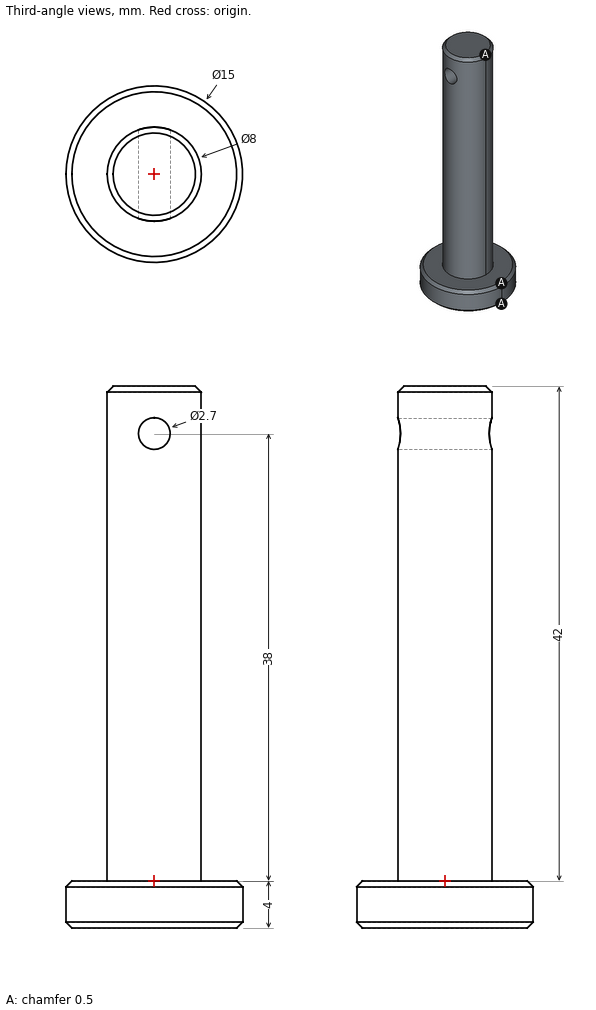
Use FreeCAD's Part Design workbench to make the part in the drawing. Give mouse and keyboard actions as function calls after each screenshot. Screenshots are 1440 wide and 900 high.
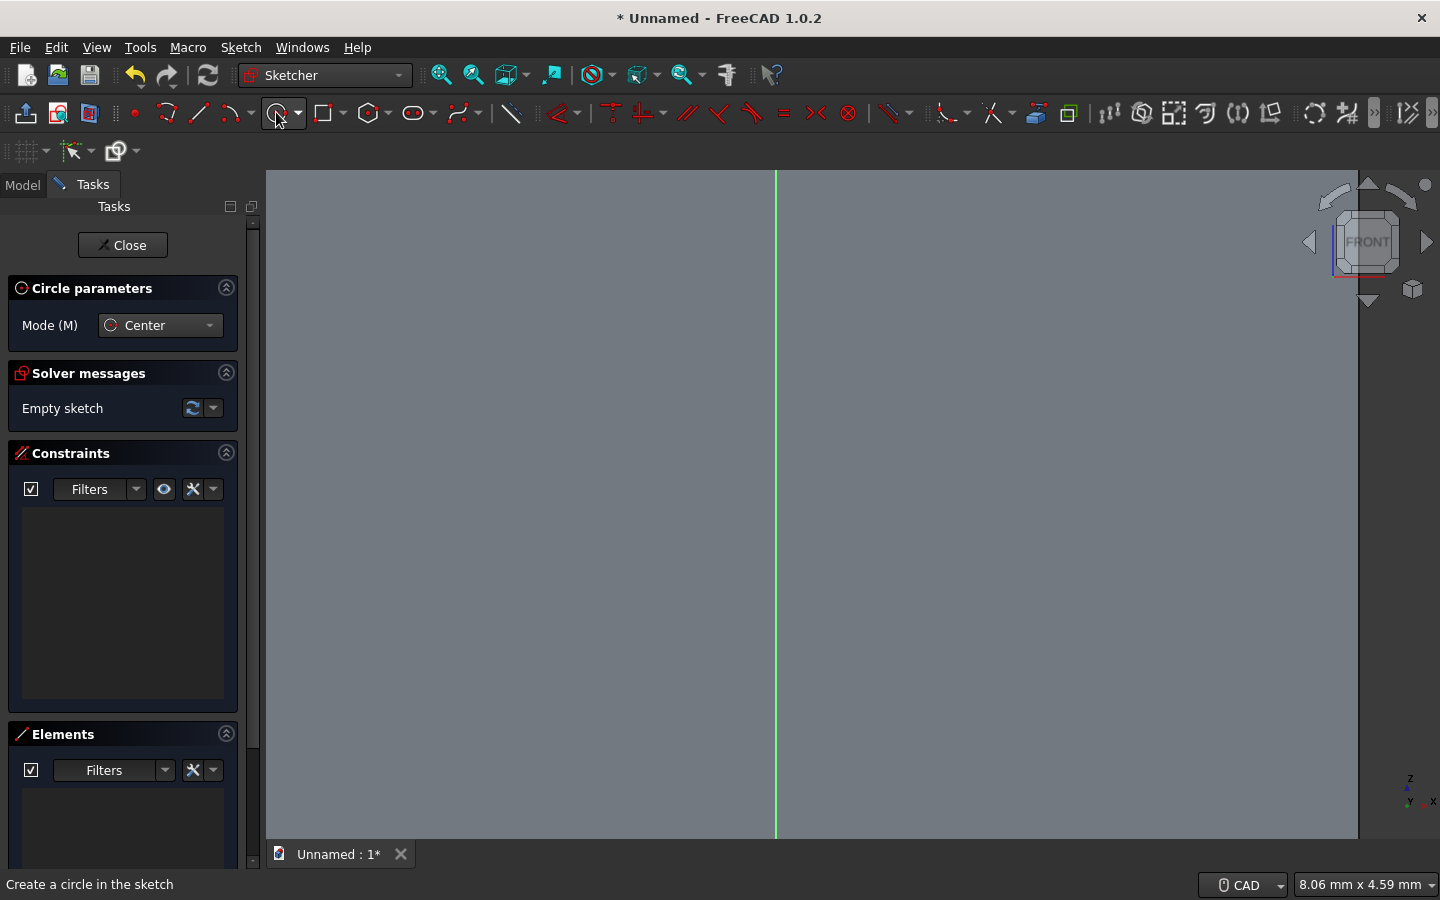
click(776, 500)
move(915, 361)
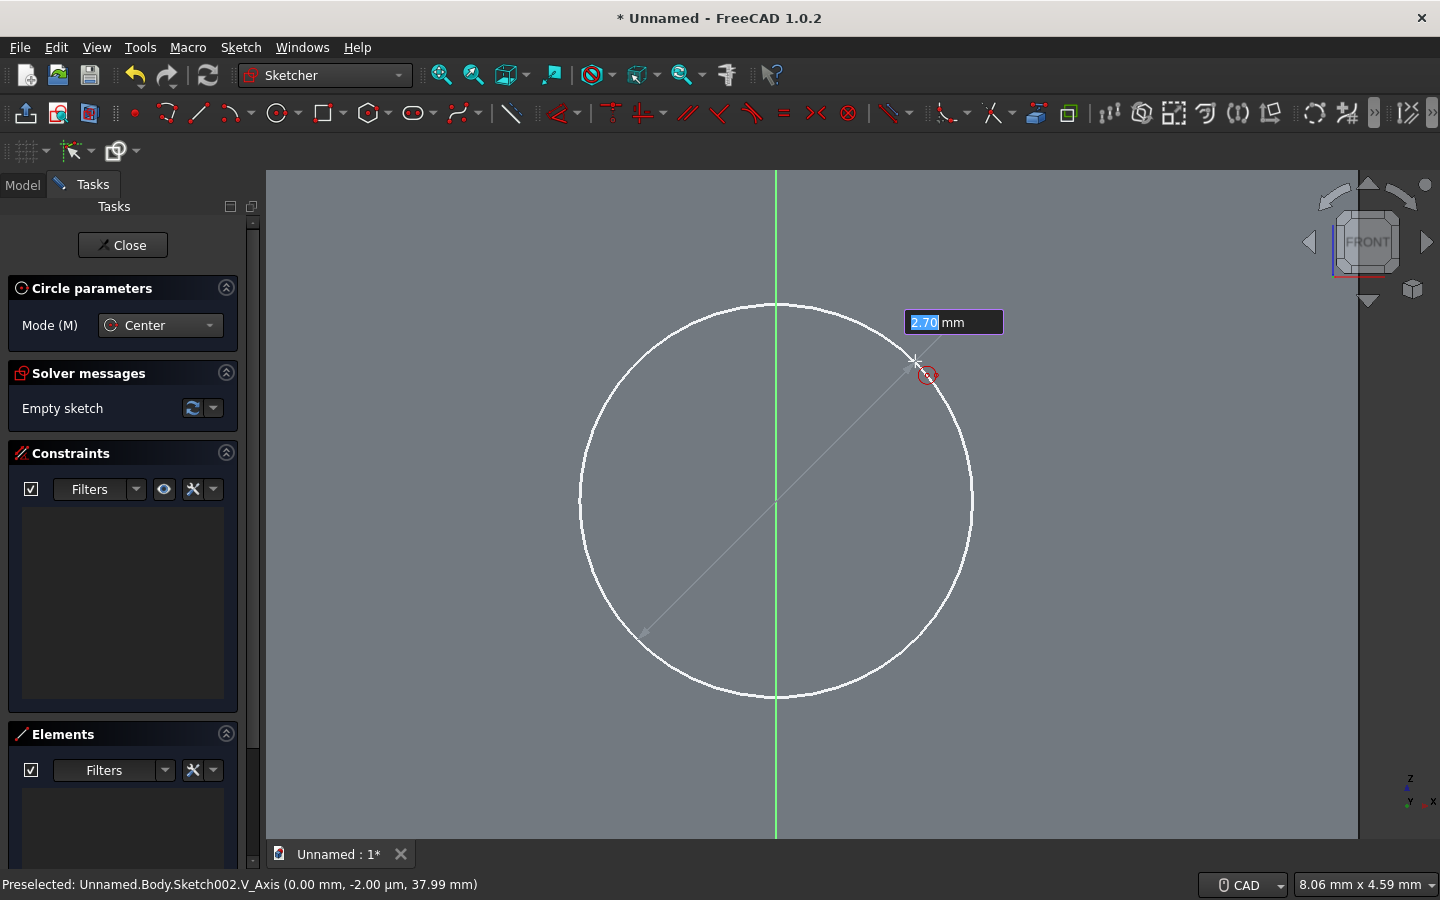
text(2.7)
key(Return)
key(Escape)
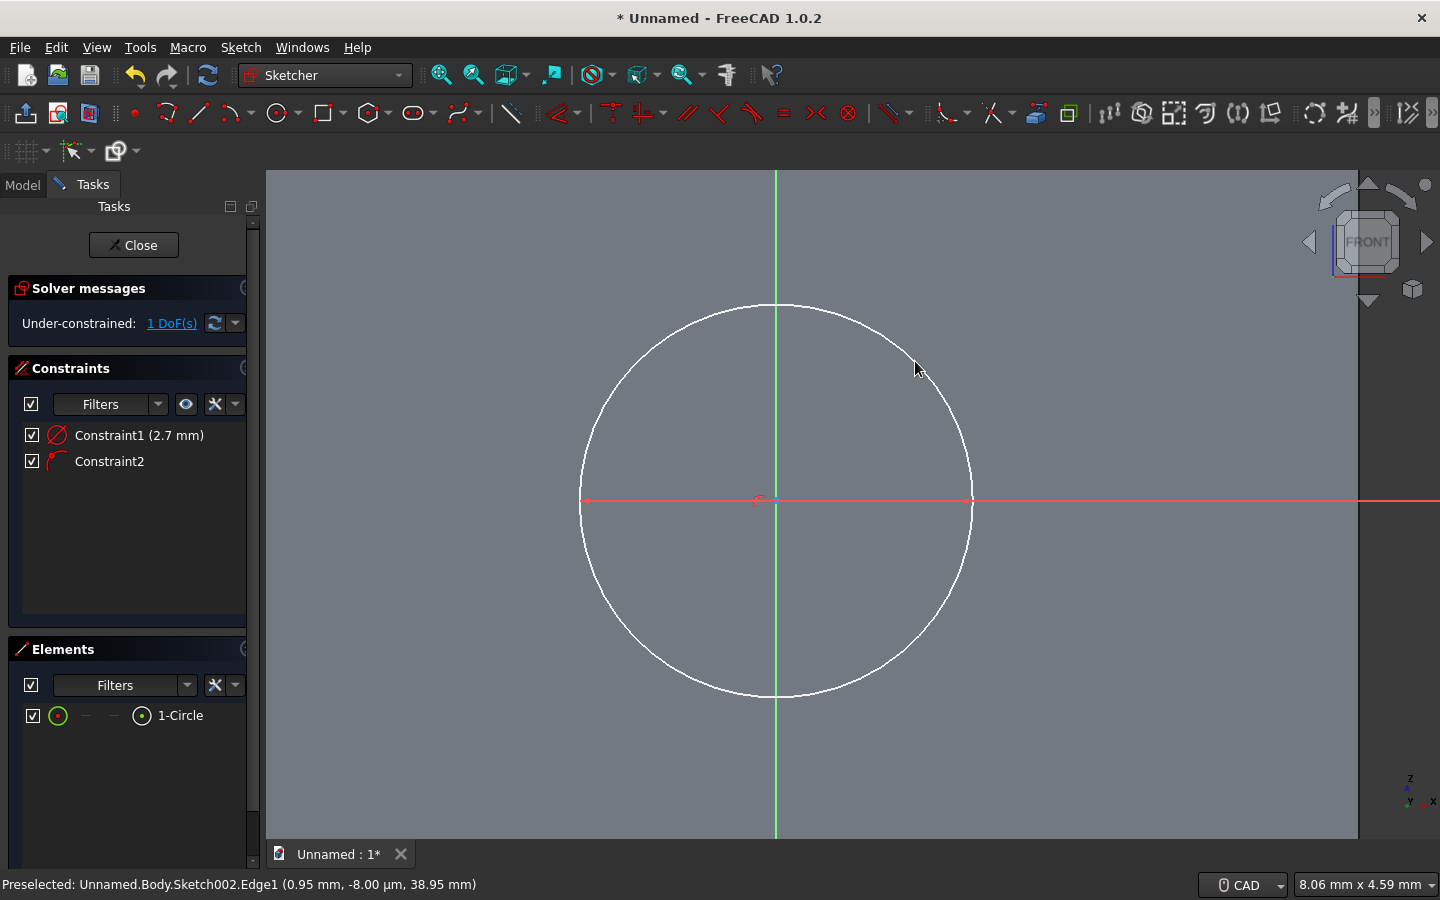
click(776, 501)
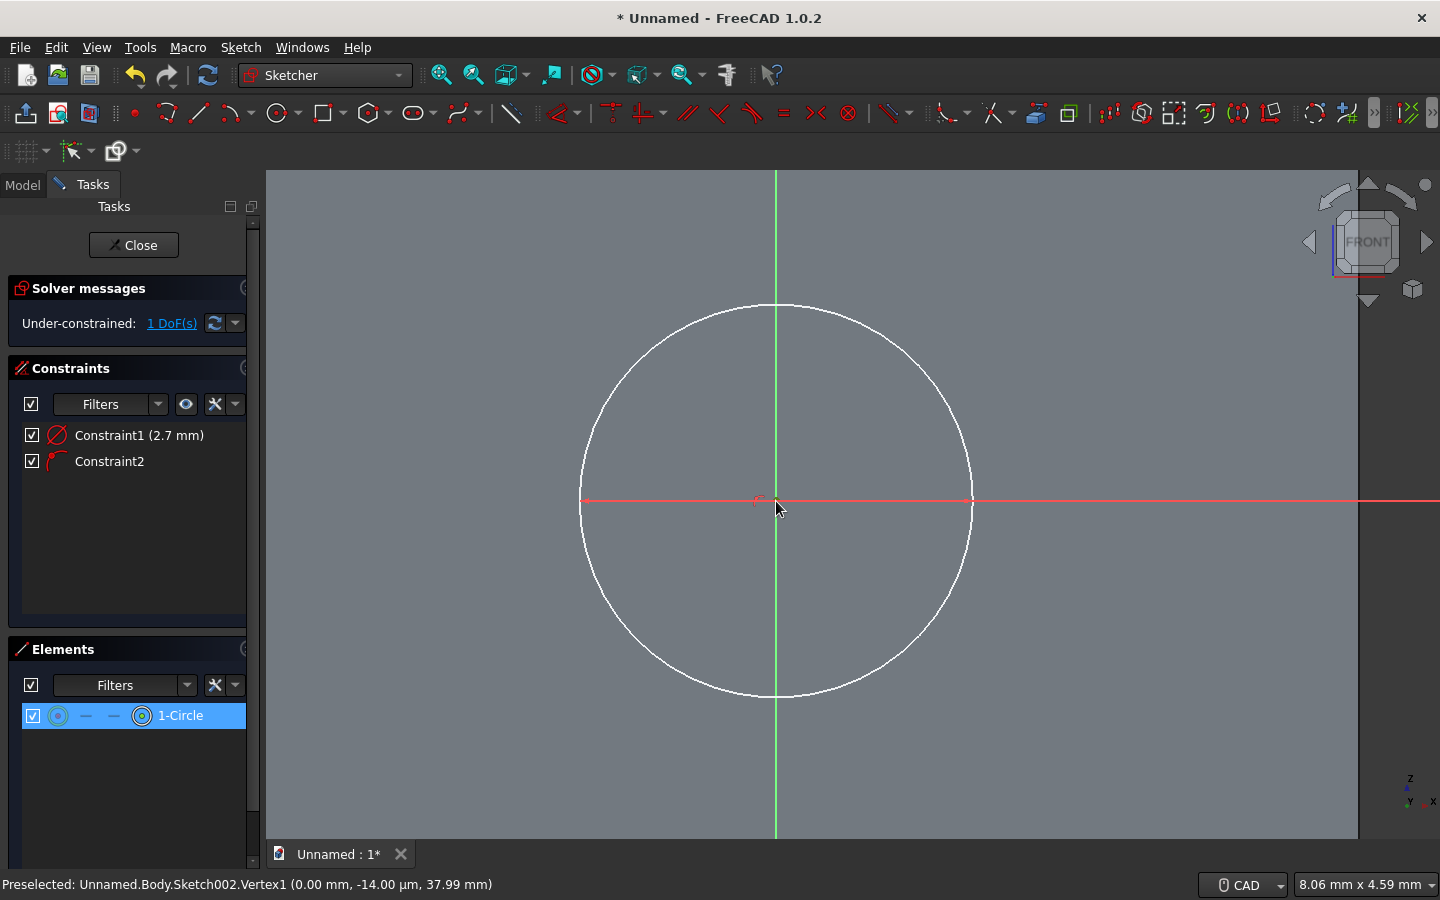
key(i)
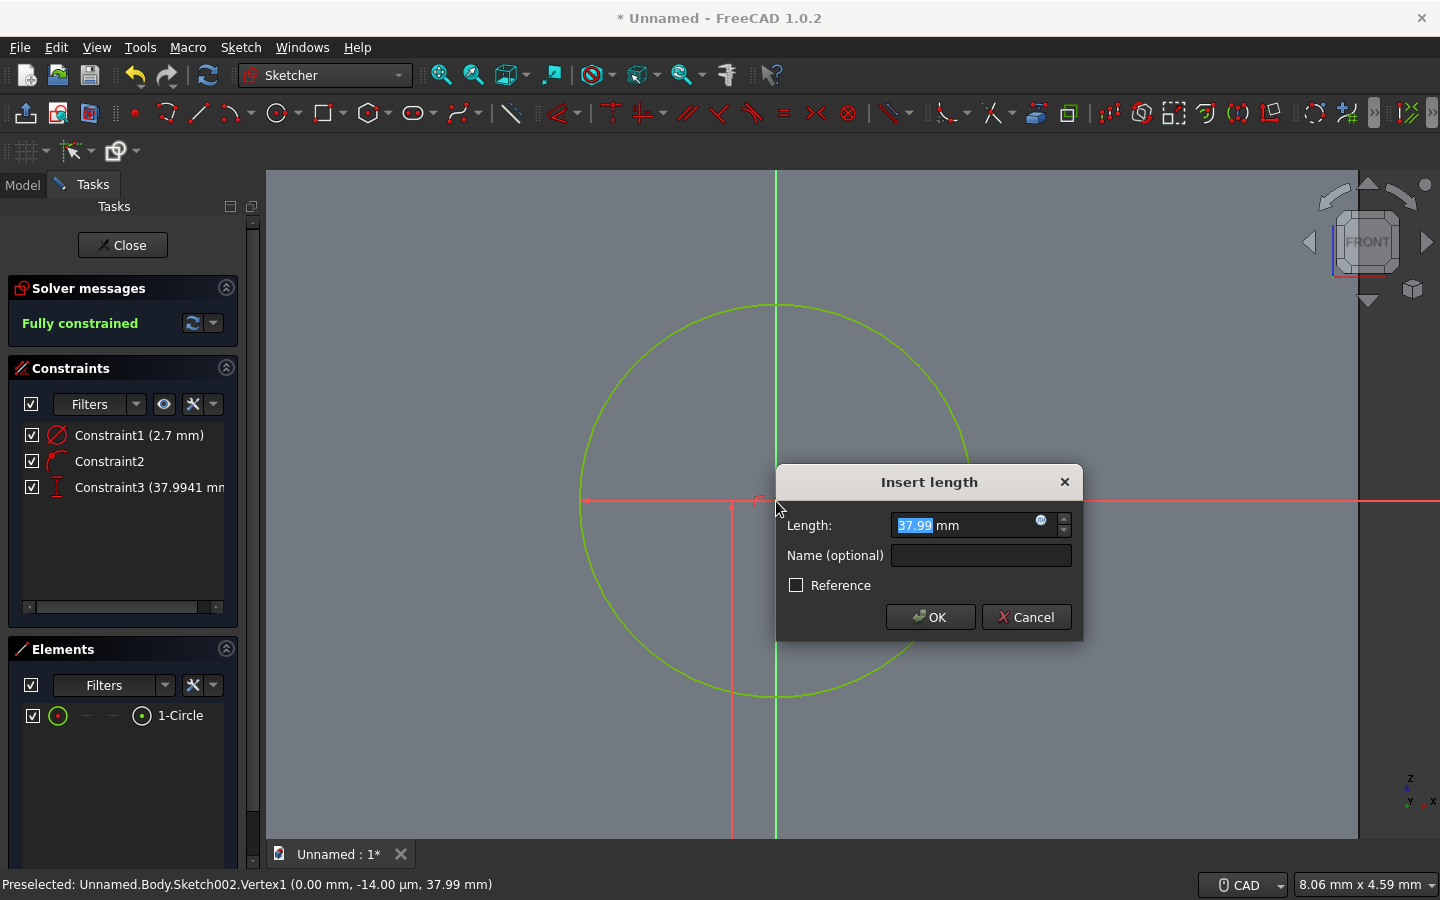
text(38)
key(Return)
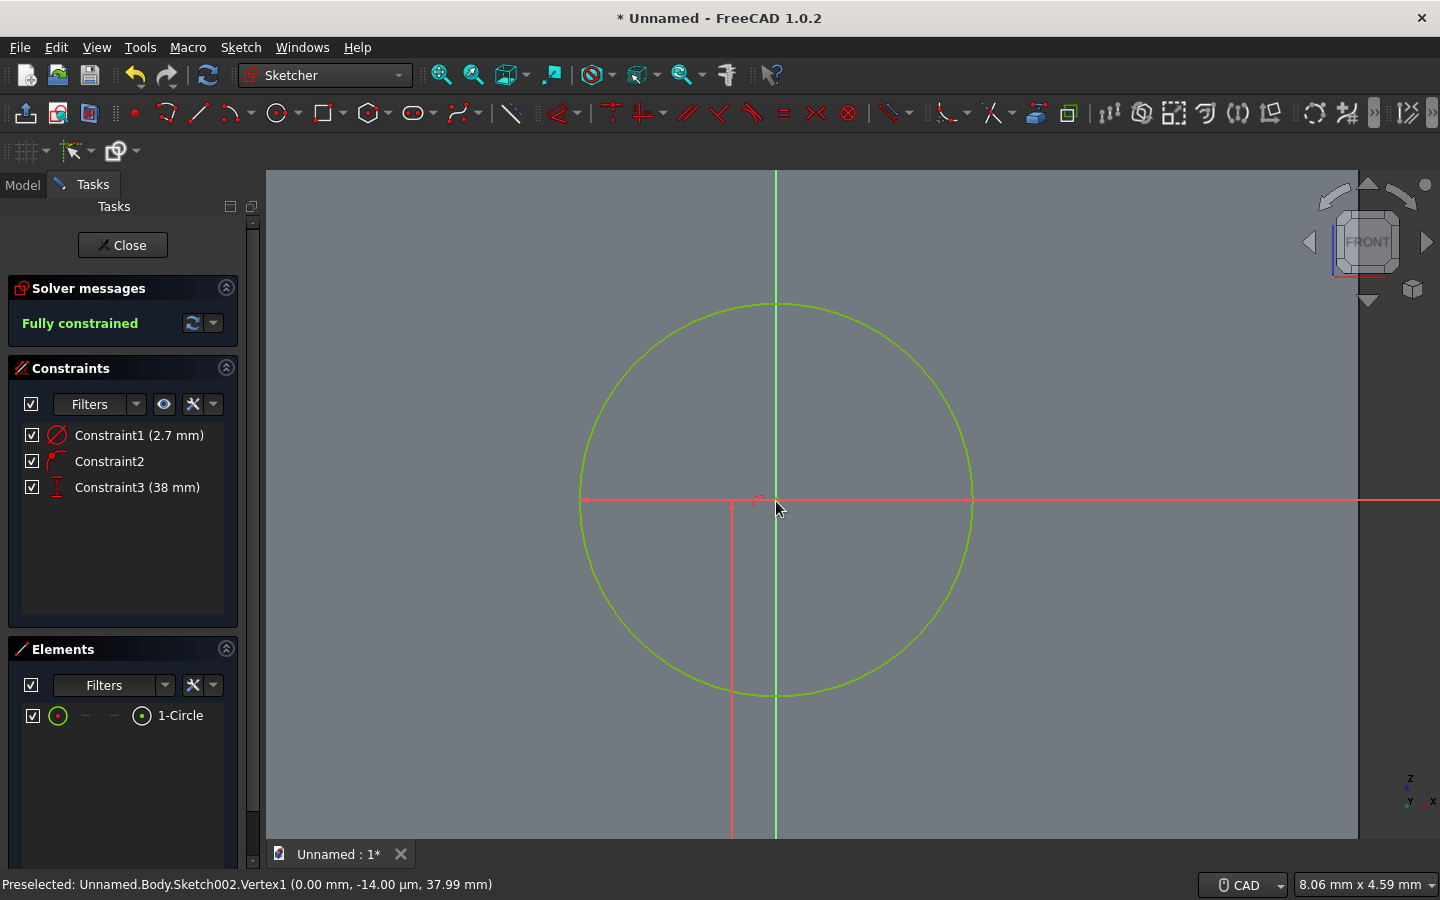
click(123, 245)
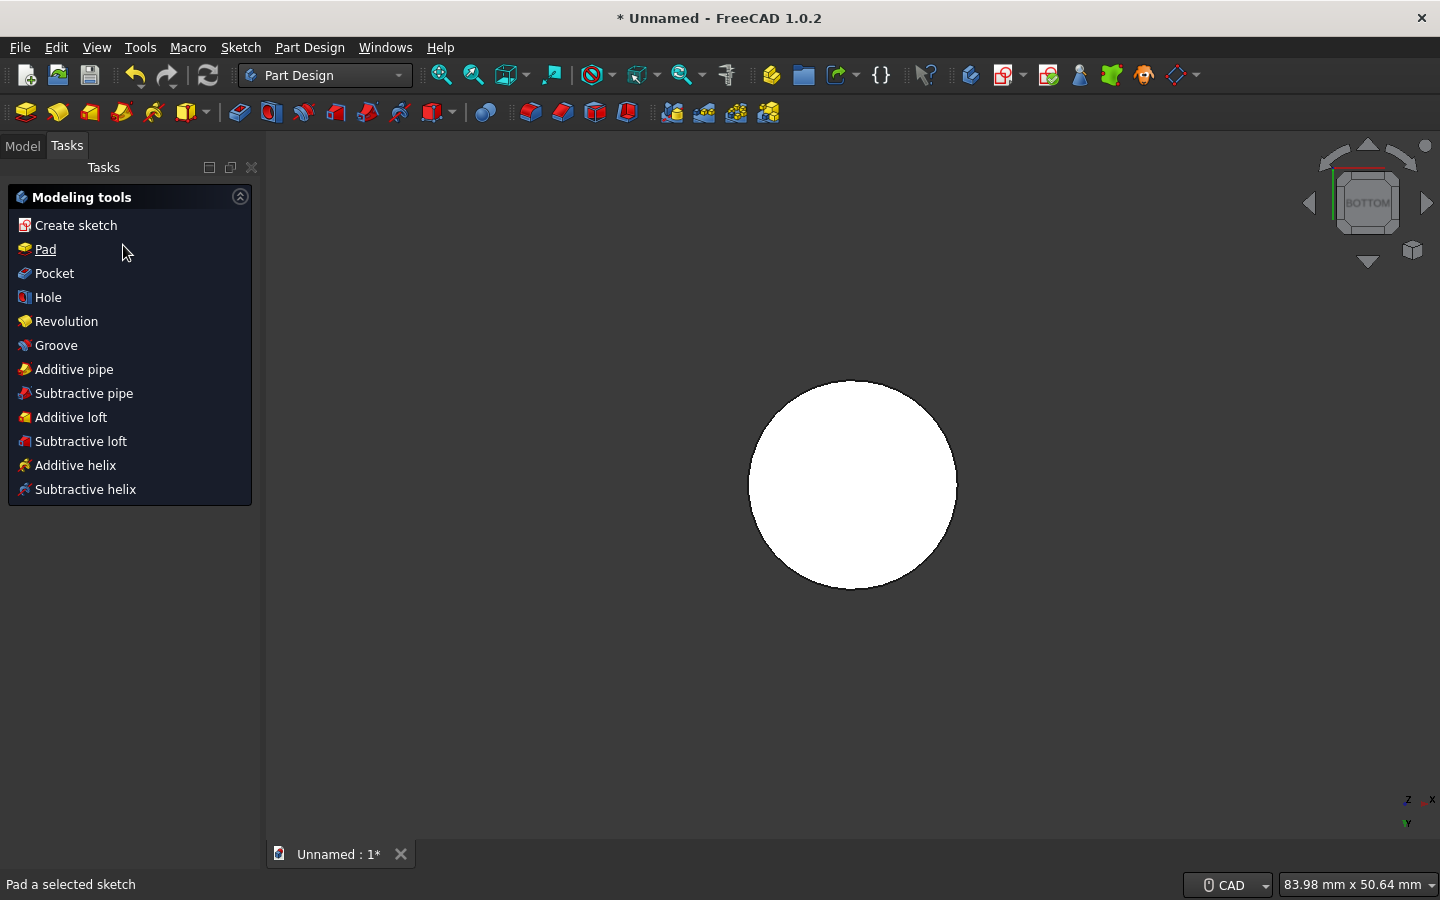
click(240, 112)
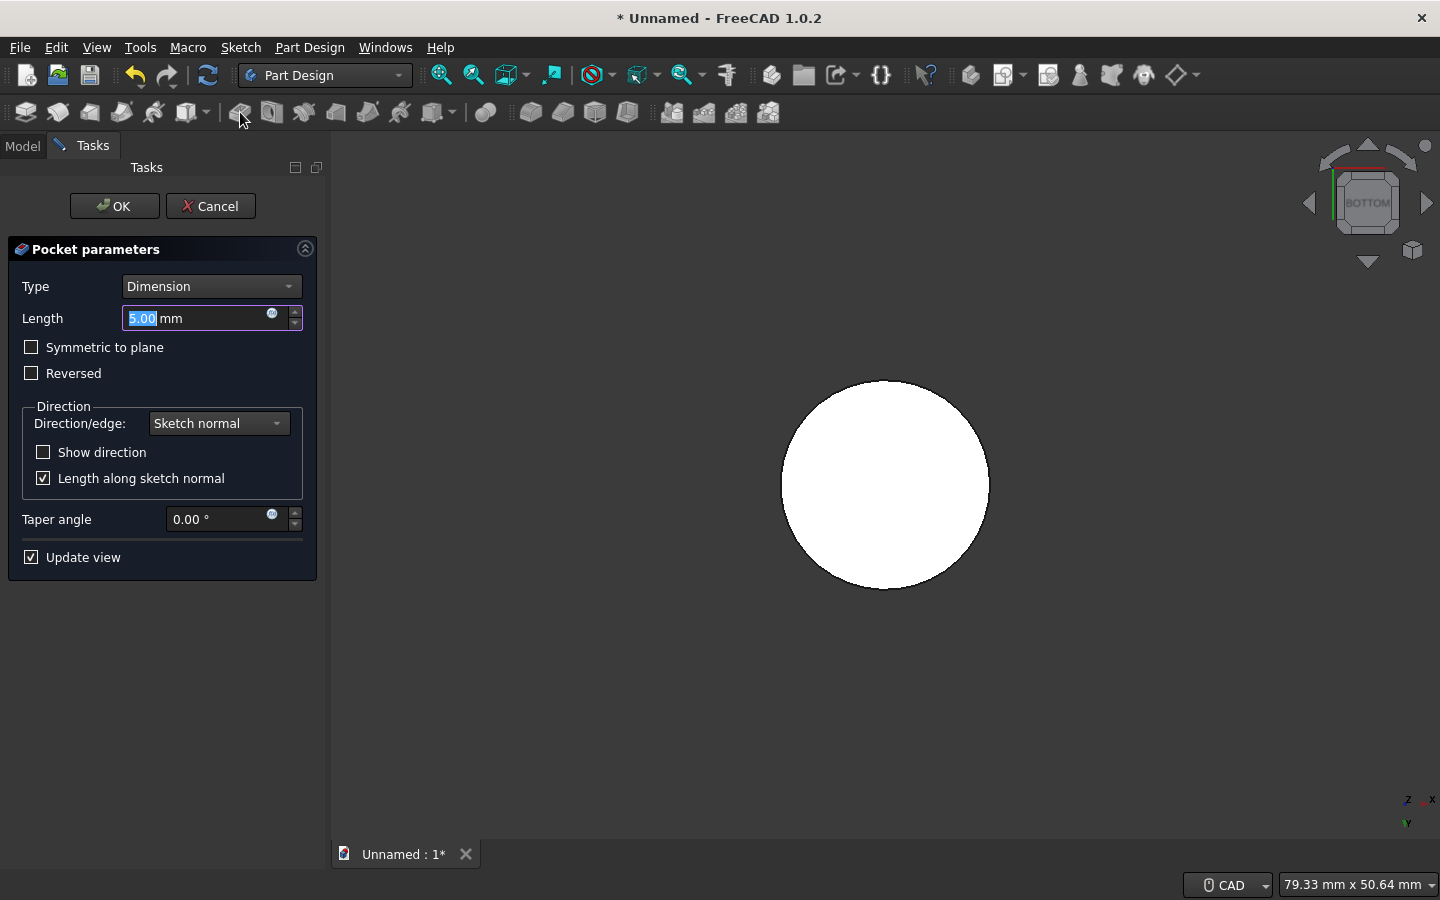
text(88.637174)
key(Tab)